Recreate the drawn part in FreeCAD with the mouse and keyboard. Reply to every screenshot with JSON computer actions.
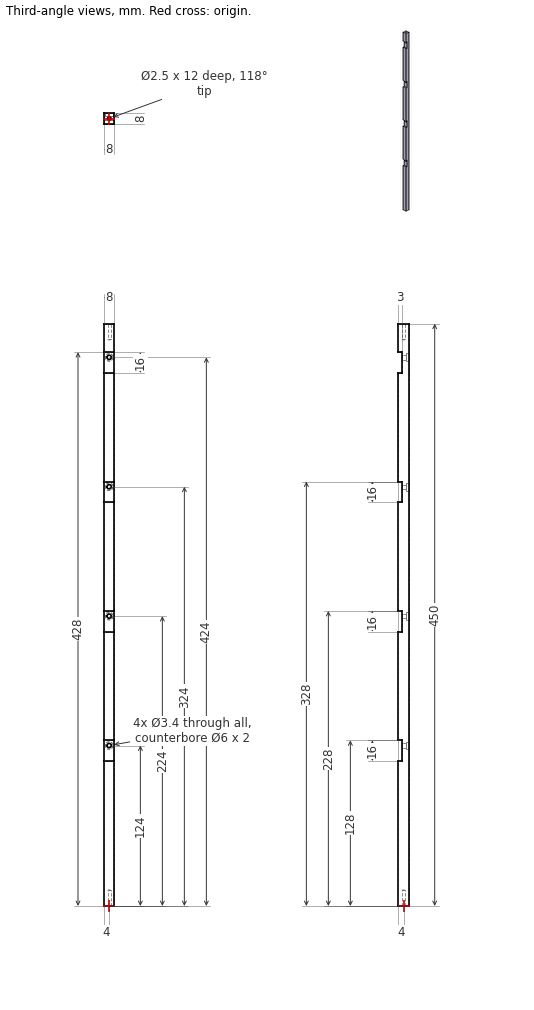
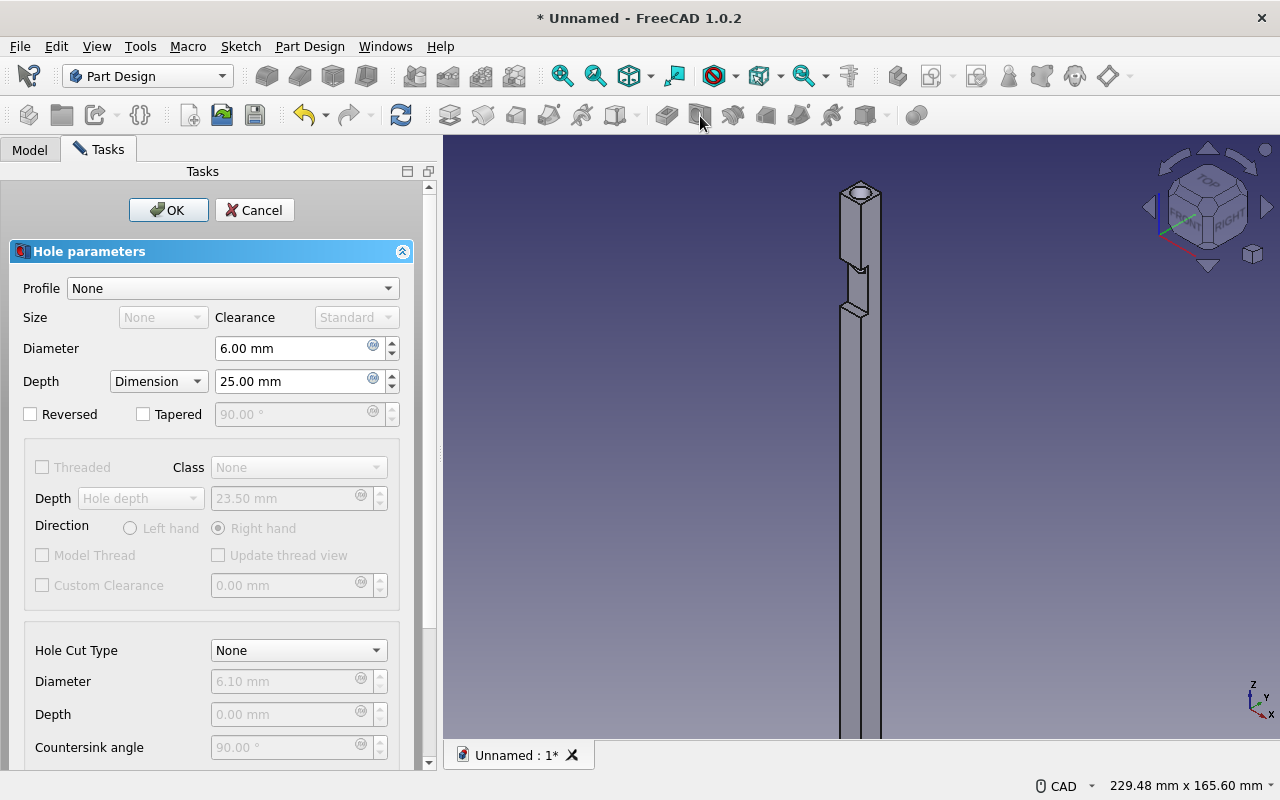
{"action": "triple_click", "coordinate": [300, 348]}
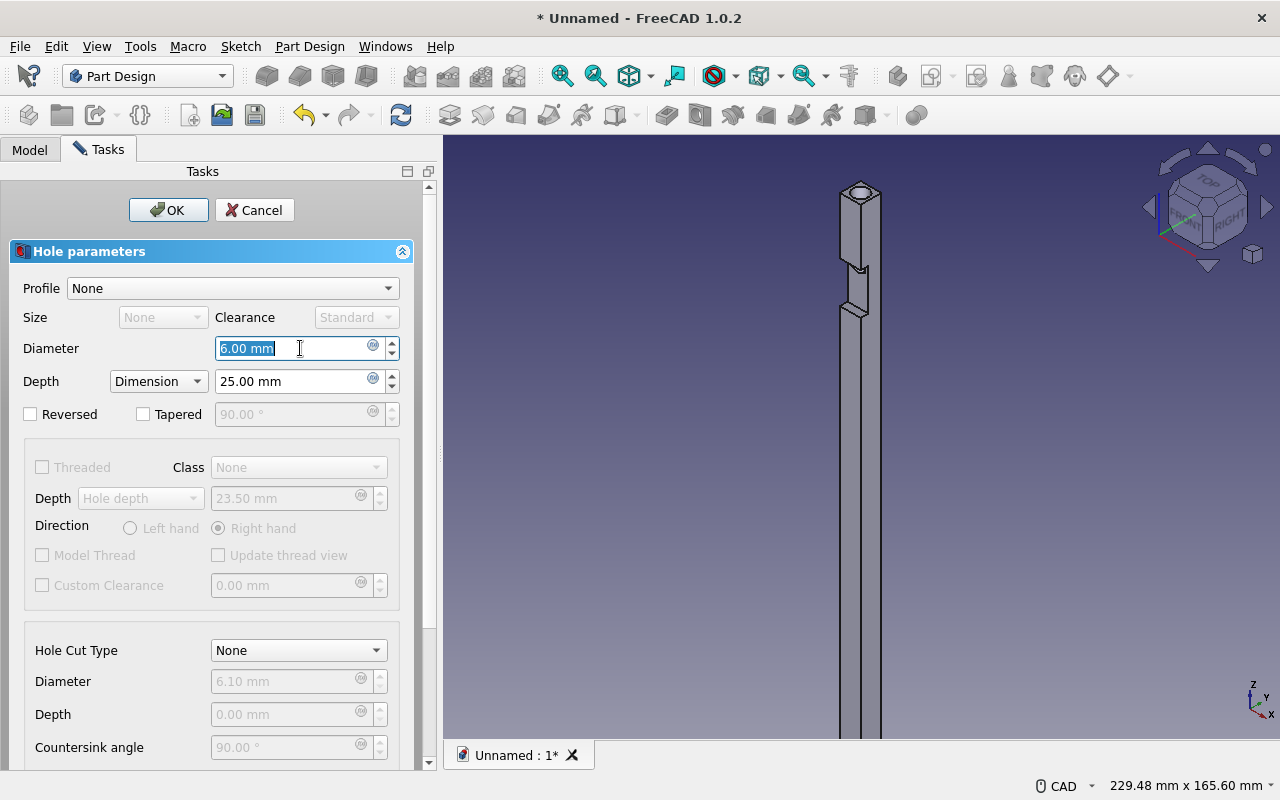
{"action": "type", "text": "2.5"}
{"action": "key", "text": "Tab"}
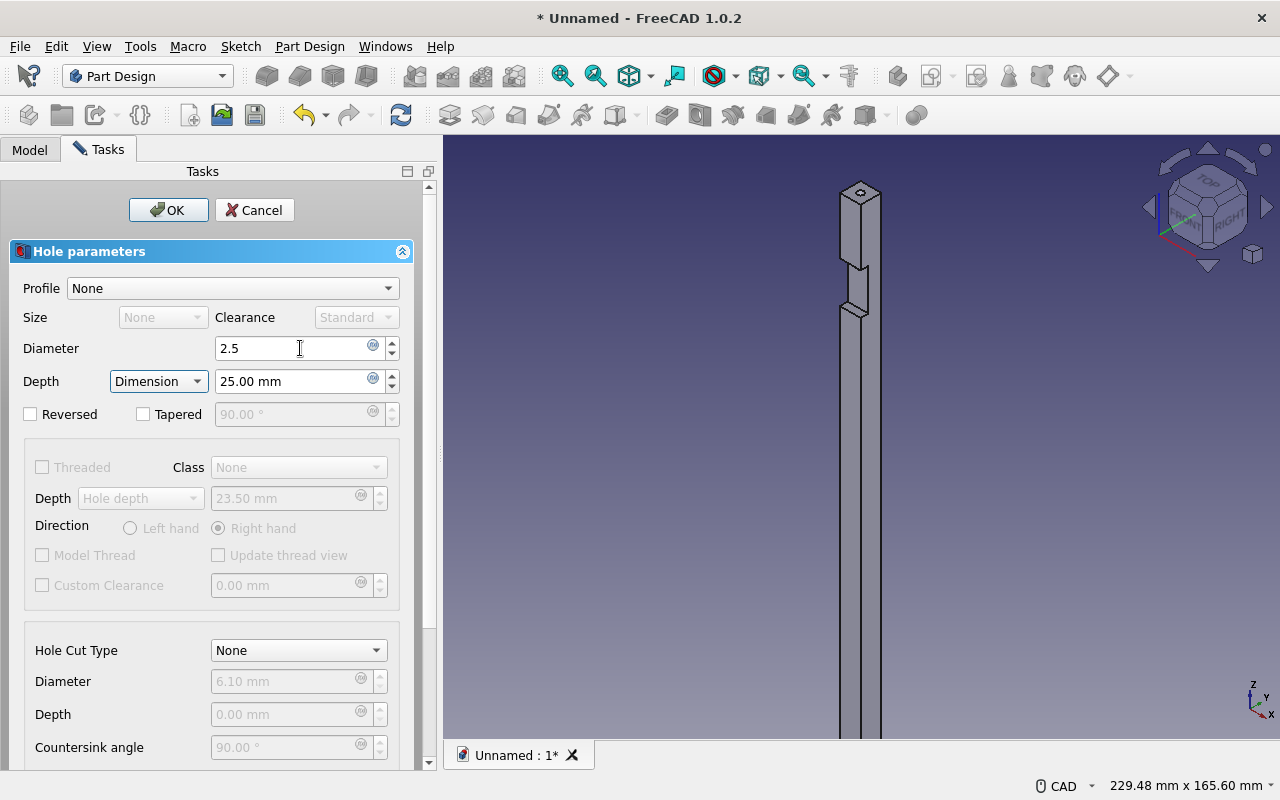
{"action": "triple_click", "coordinate": [300, 382]}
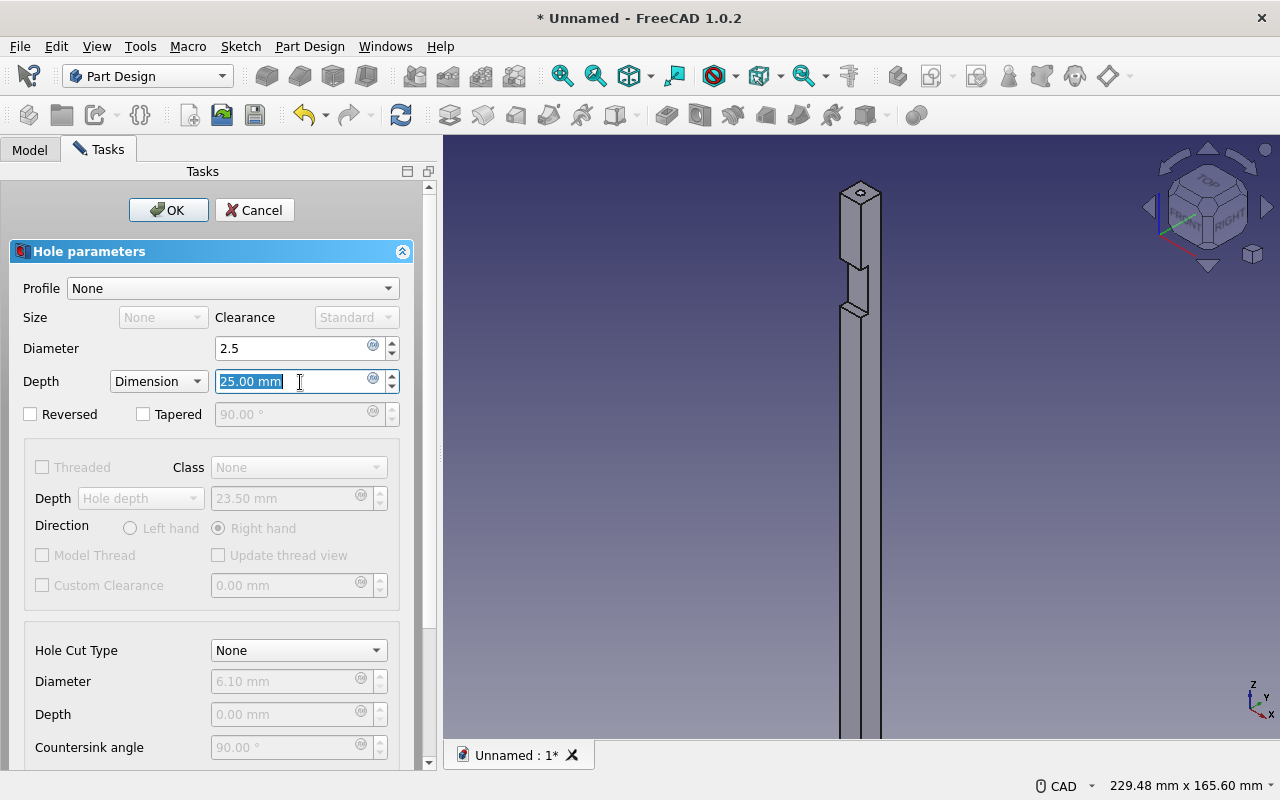
{"action": "type", "text": "12"}
{"action": "key", "text": "Tab"}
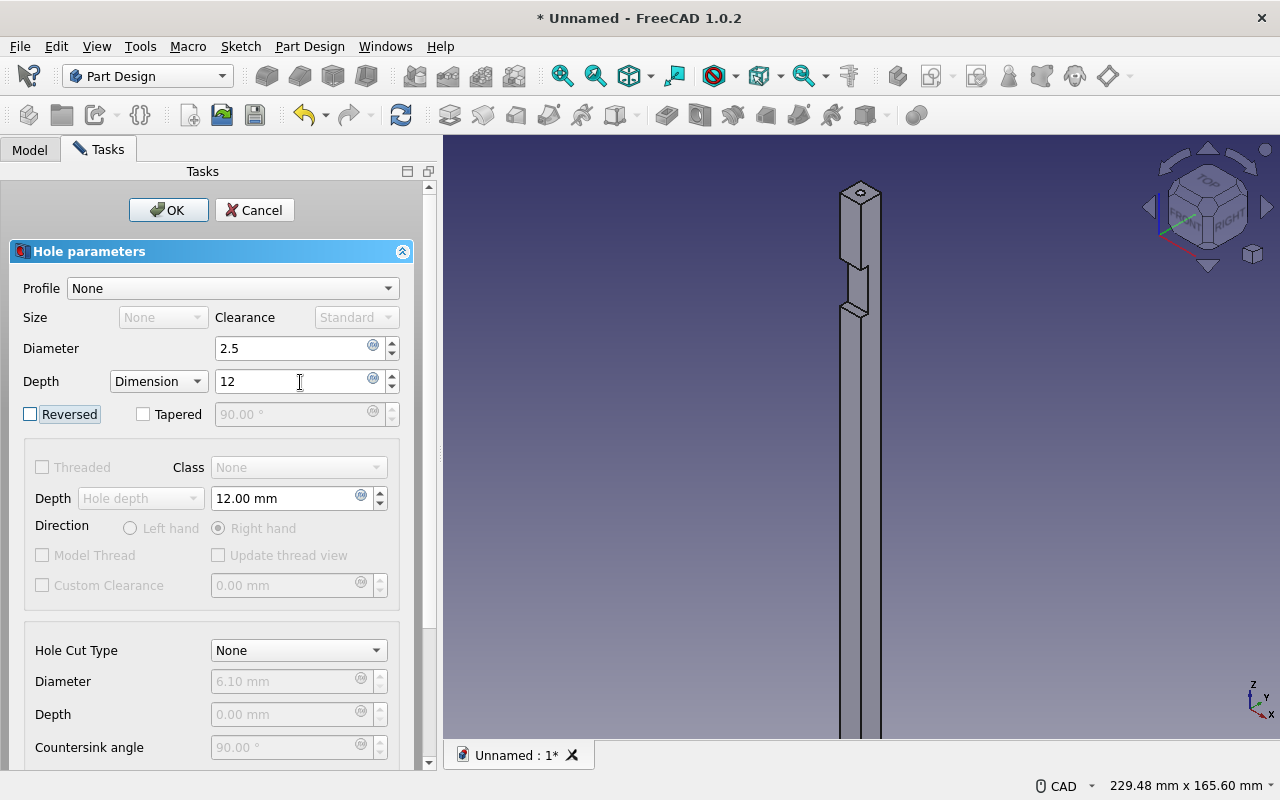
{"action": "left_click", "coordinate": [169, 210]}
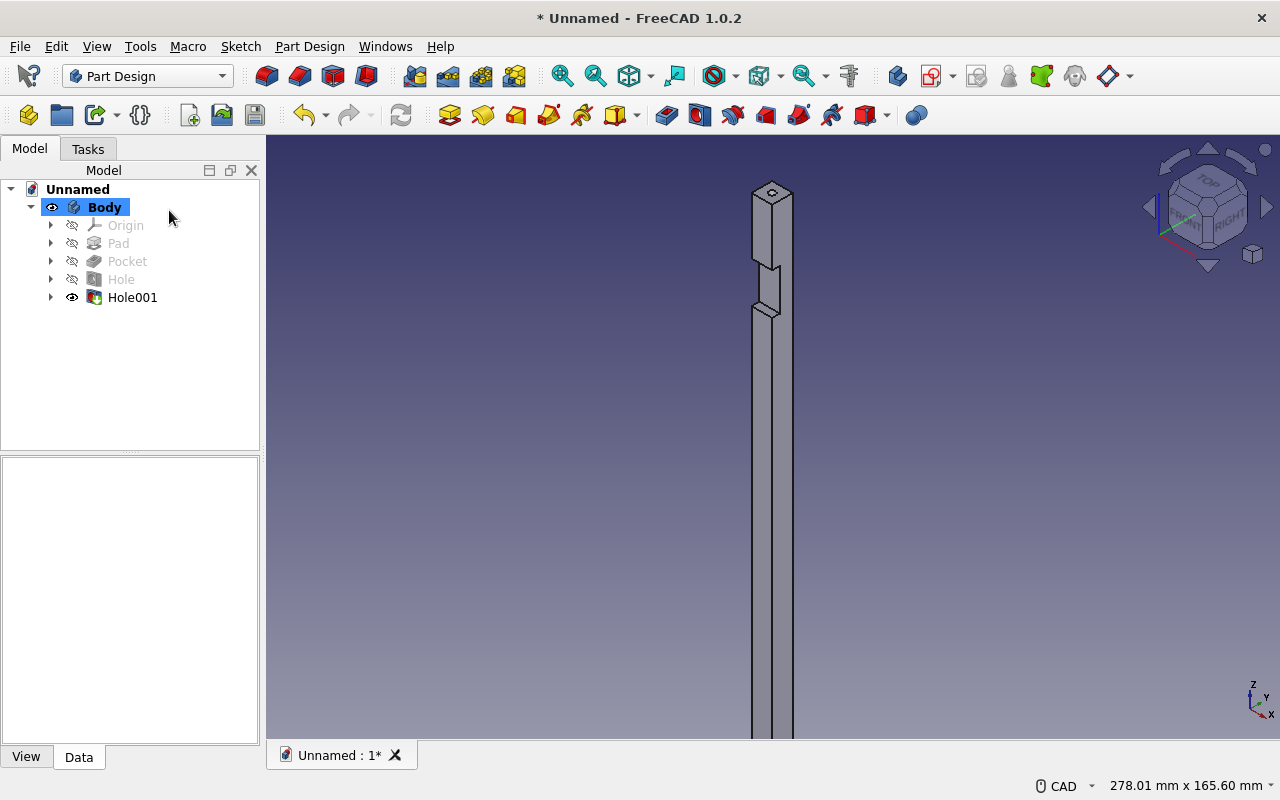
{"action": "key", "text": "v f"}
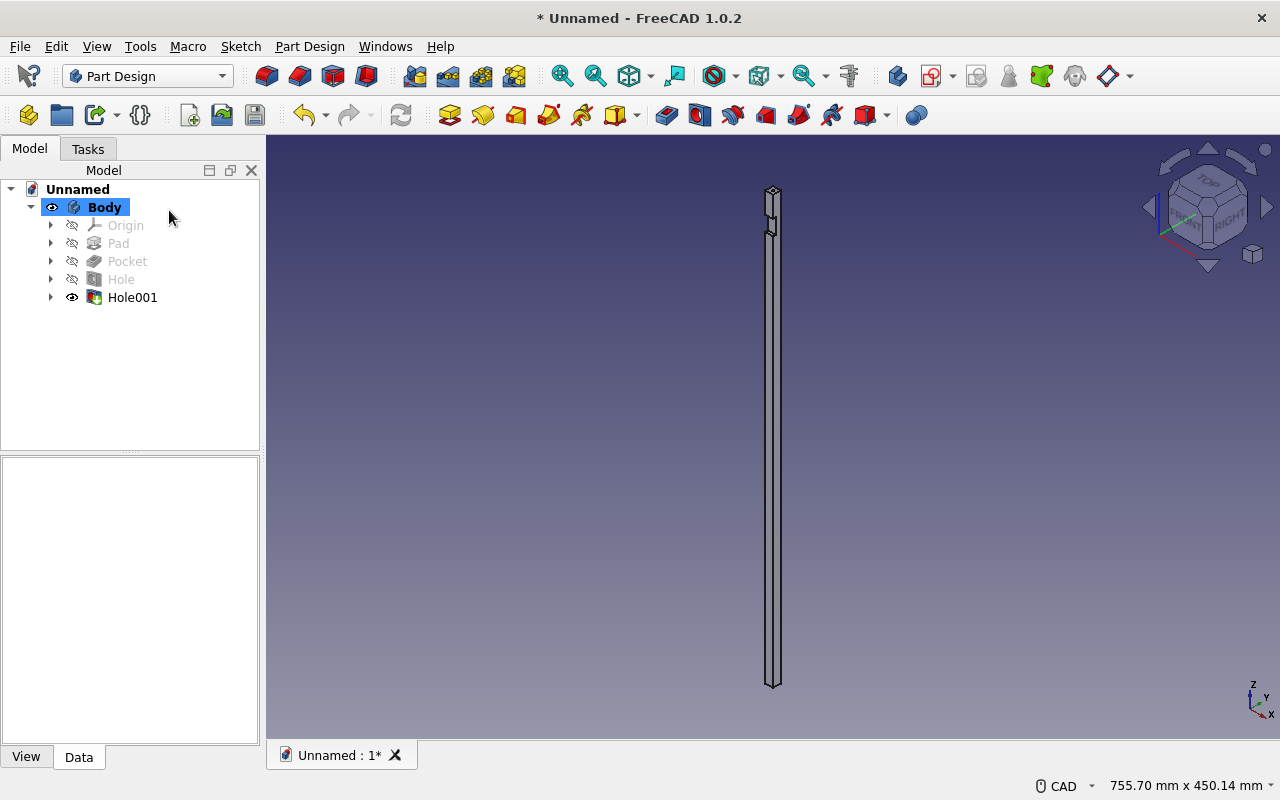
{"action": "scroll", "coordinate": [777, 297], "scroll_direction": "up", "scroll_amount": 5}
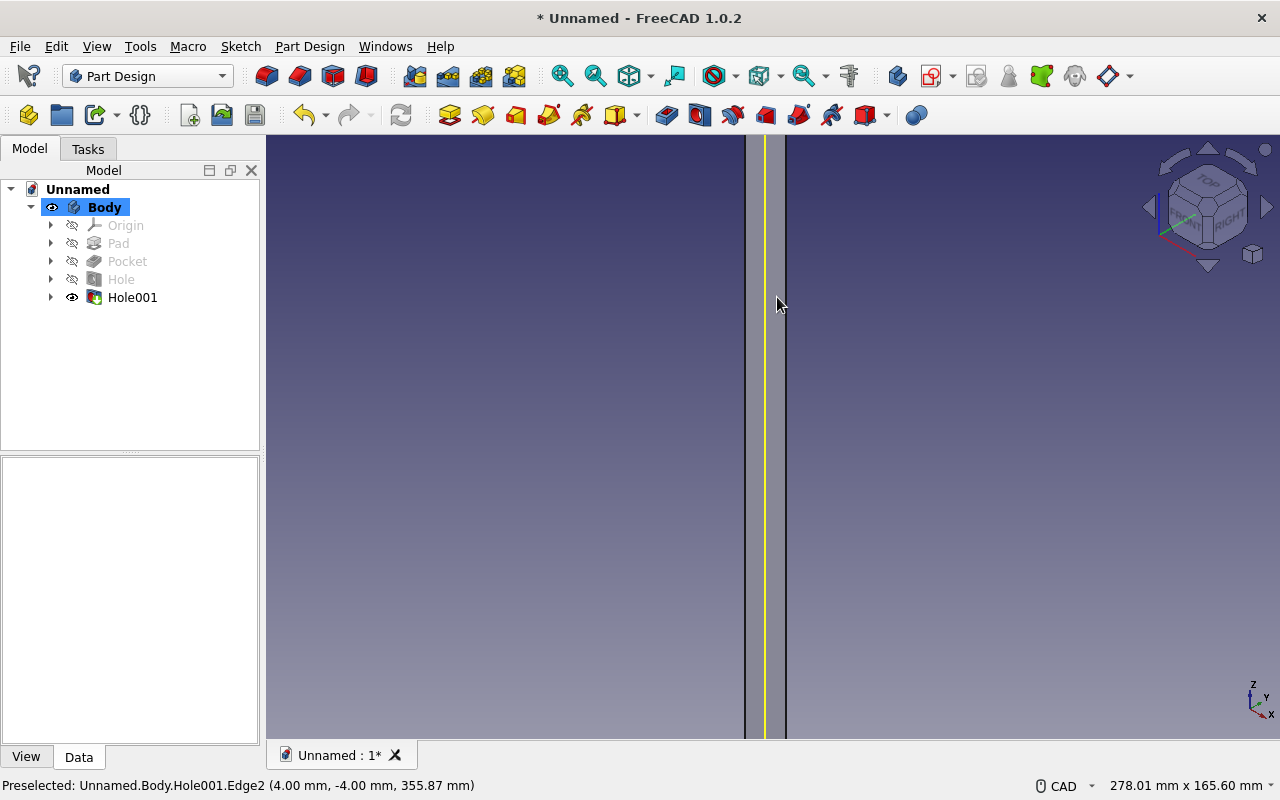
{"action": "left_click", "coordinate": [776, 299]}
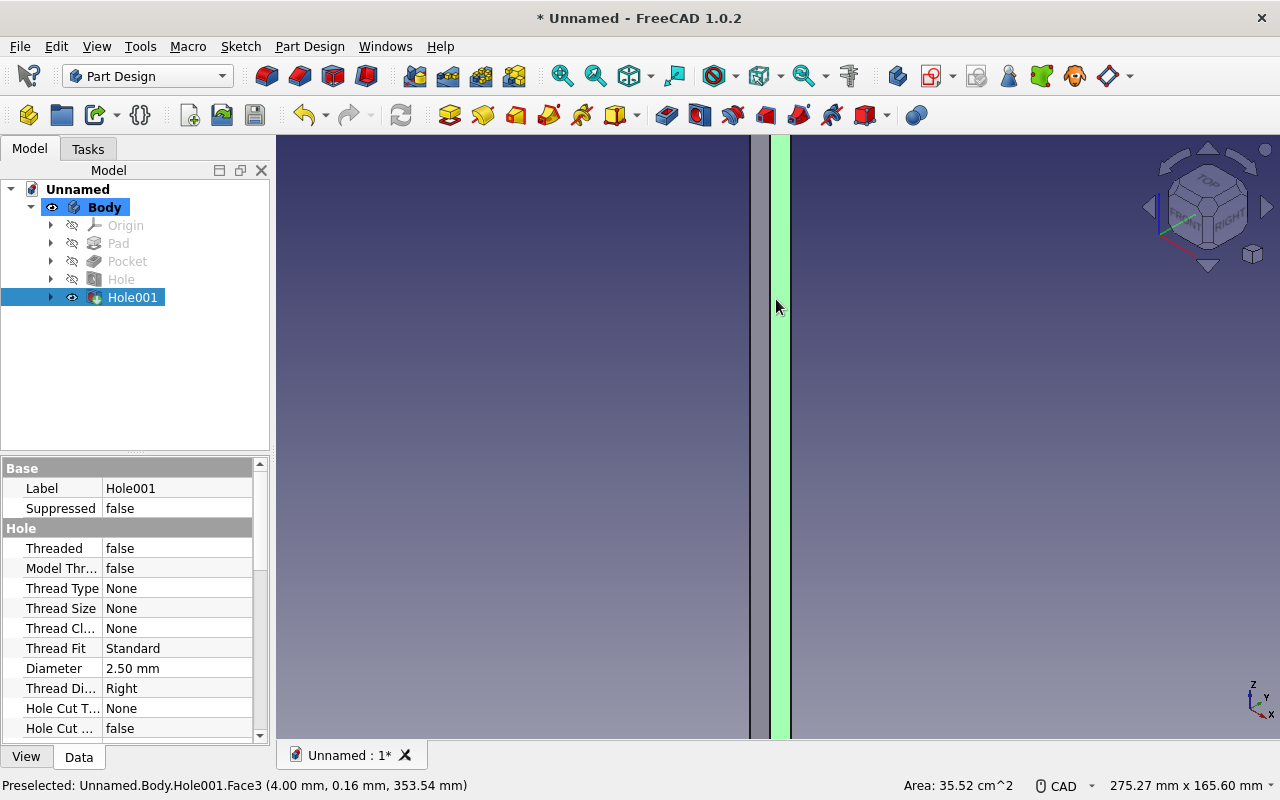
{"action": "left_click", "coordinate": [930, 76]}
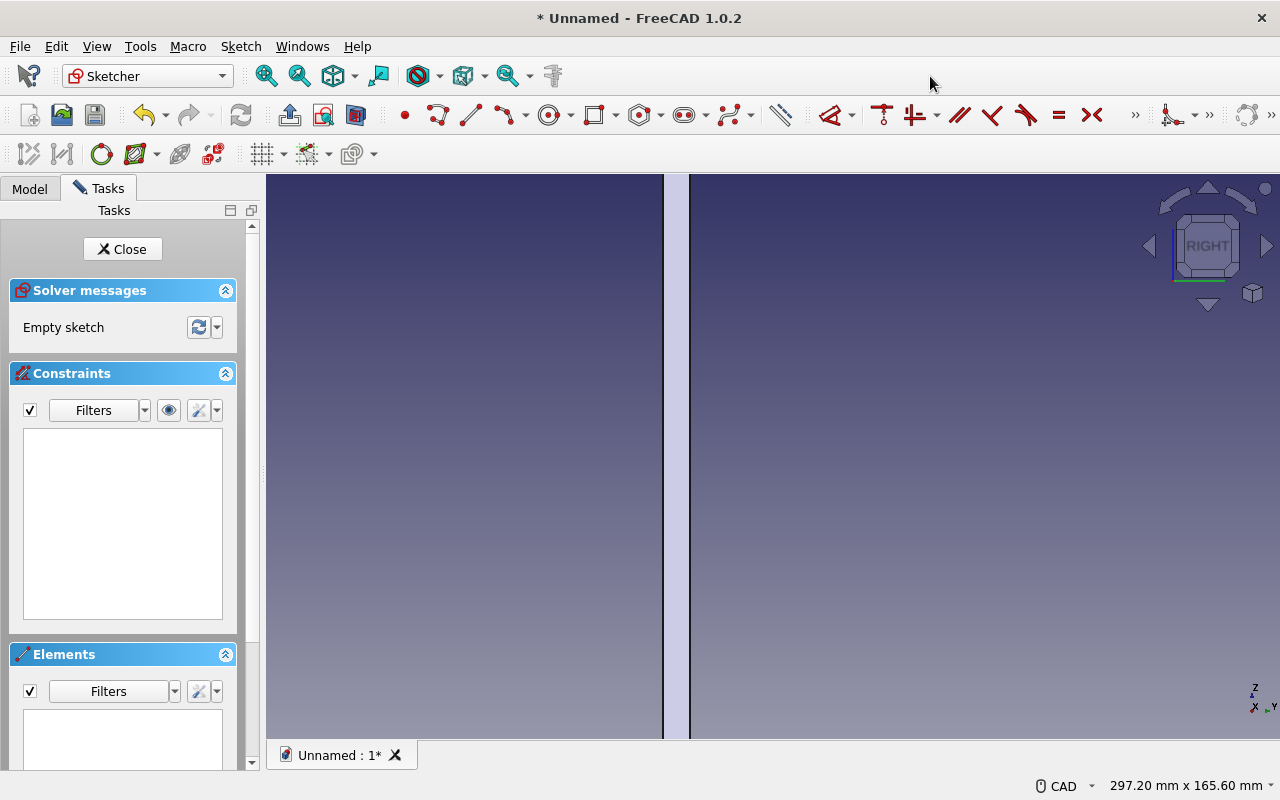
{"action": "scroll", "coordinate": [720, 288], "scroll_direction": "down", "scroll_amount": 6}